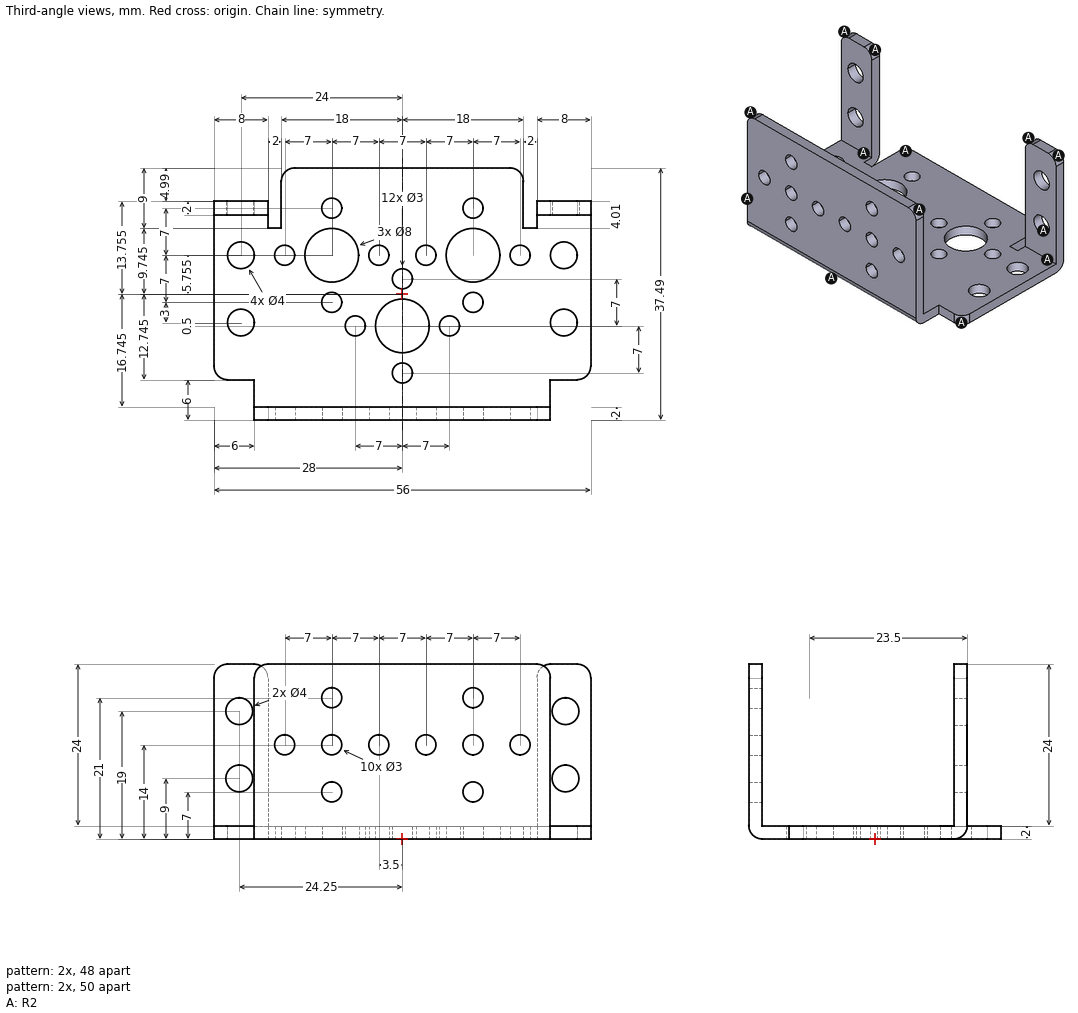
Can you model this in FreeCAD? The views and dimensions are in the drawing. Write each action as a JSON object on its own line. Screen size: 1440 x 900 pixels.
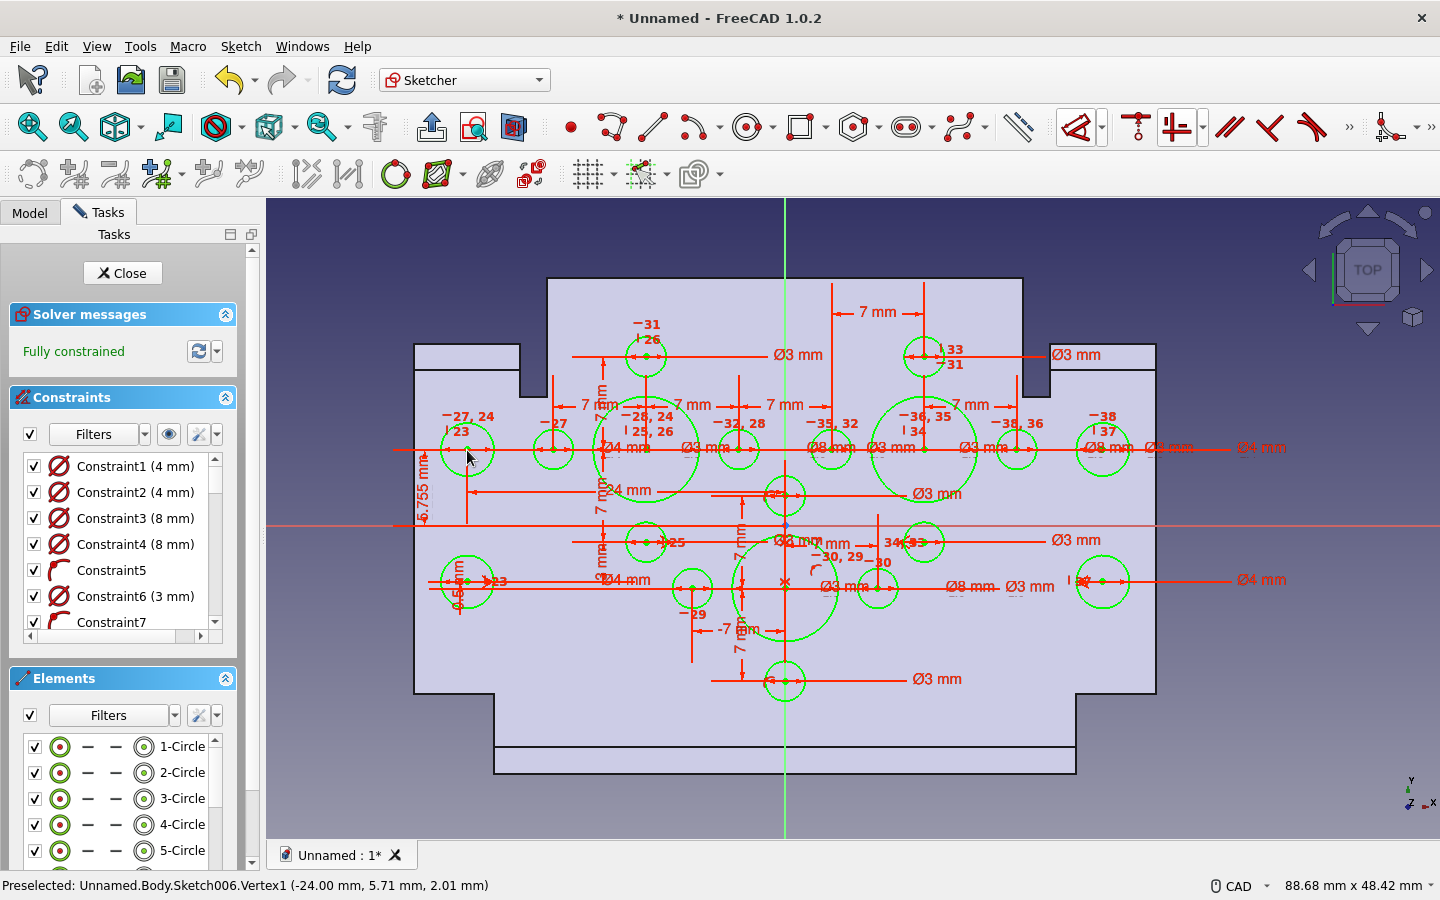
{"action": "left_click", "coordinate": [123, 273]}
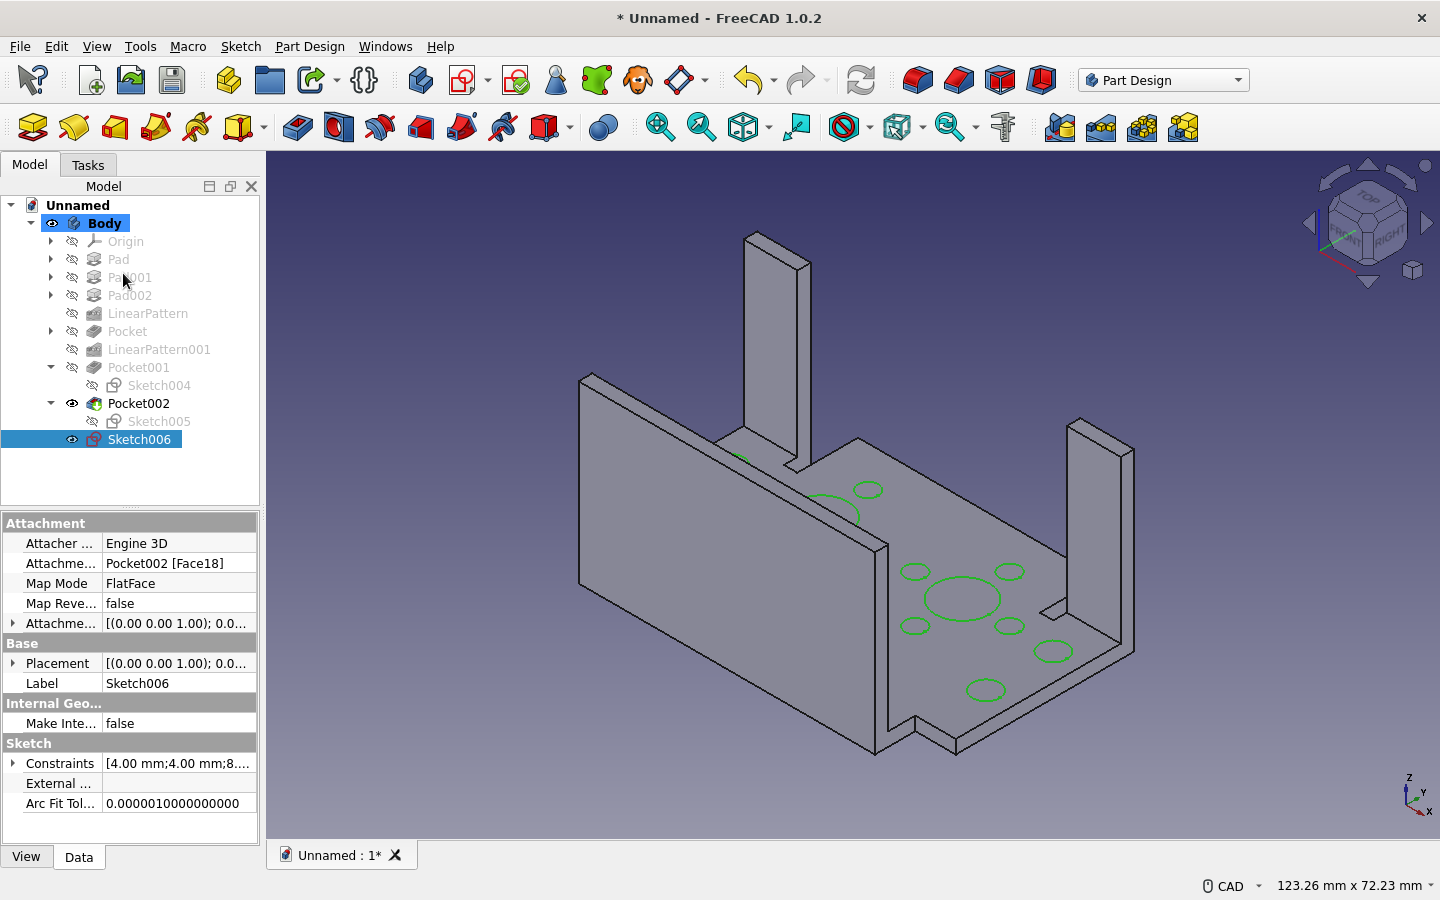
{"action": "left_click", "coordinate": [298, 128]}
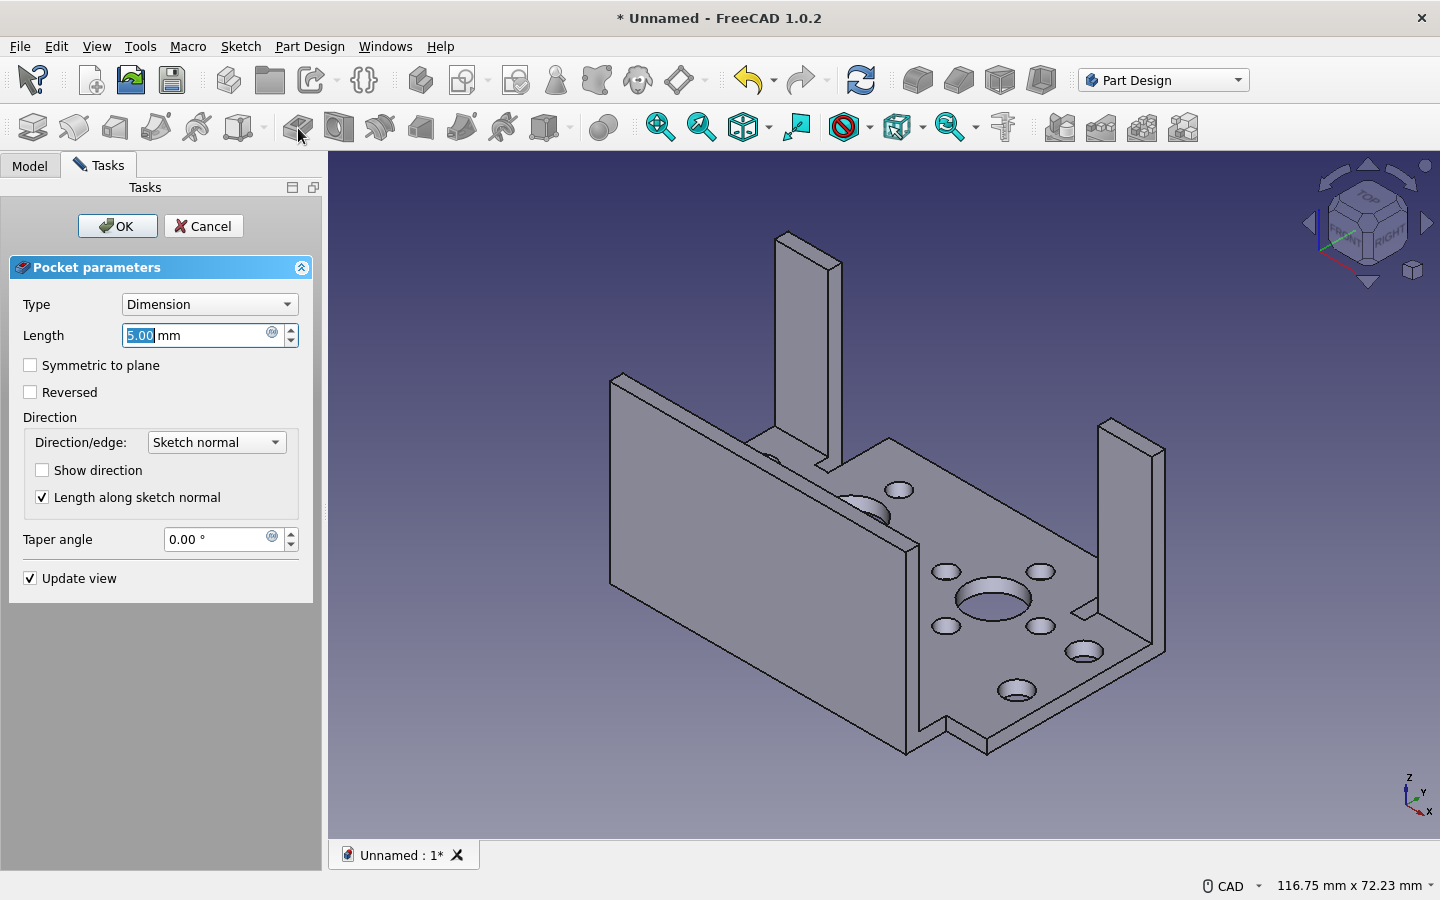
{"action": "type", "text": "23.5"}
{"action": "key", "text": "Tab"}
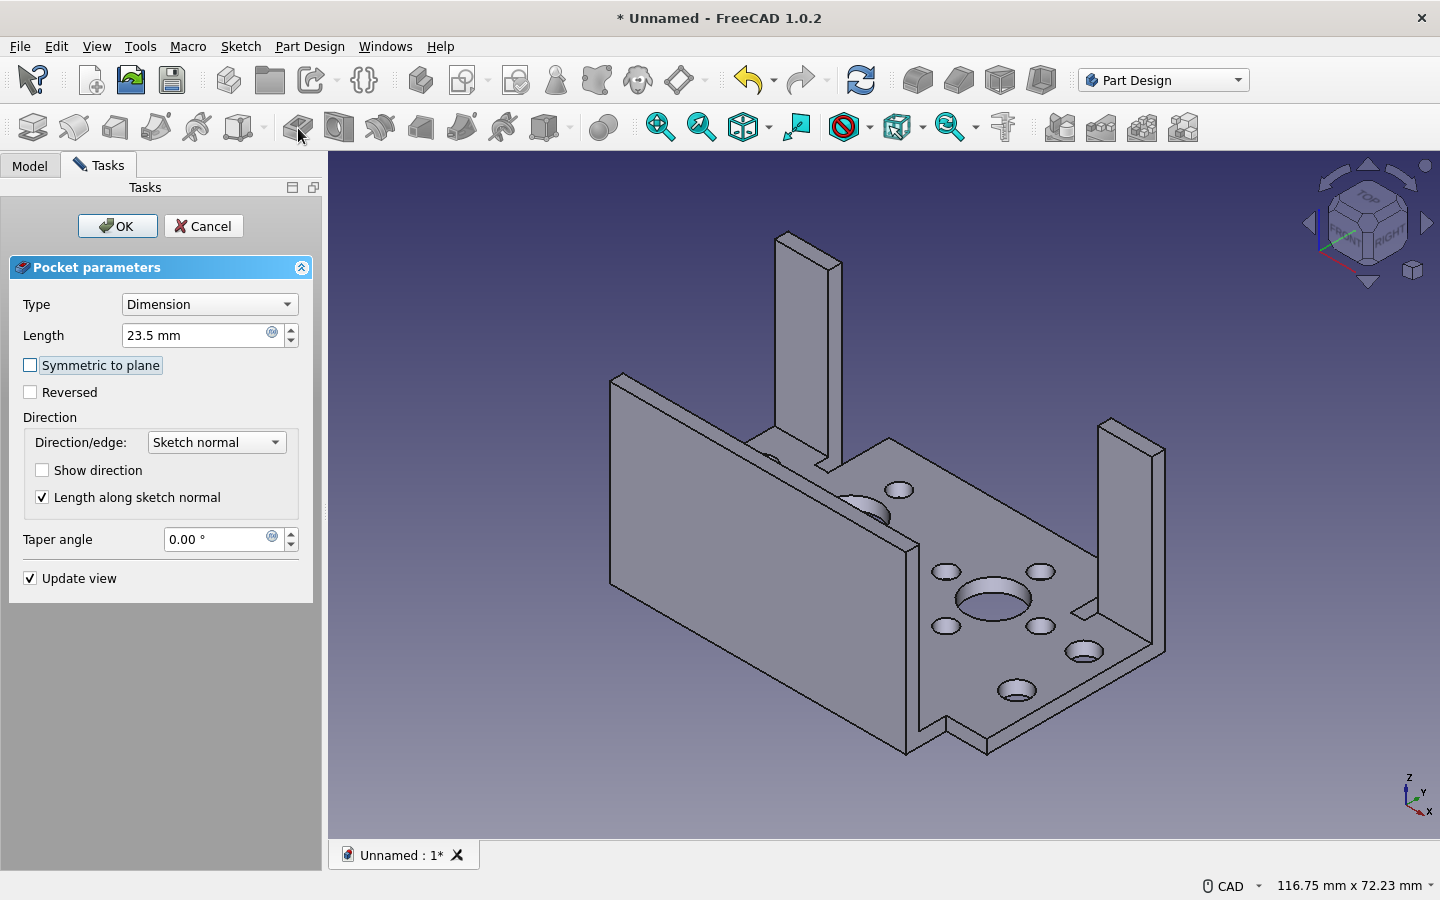
{"action": "left_click", "coordinate": [118, 226]}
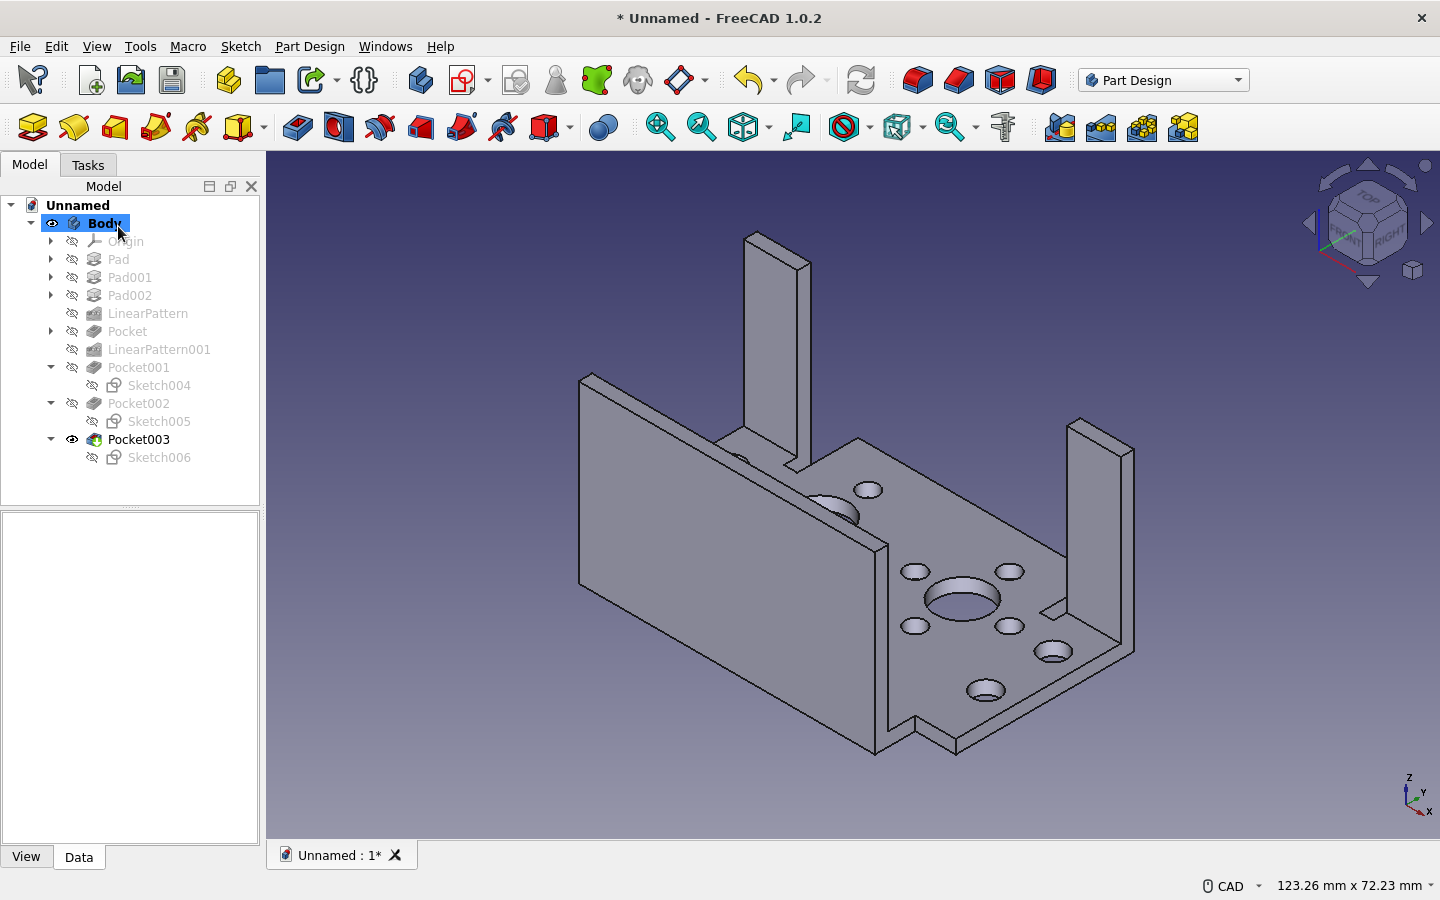
{"action": "key", "text": "4"}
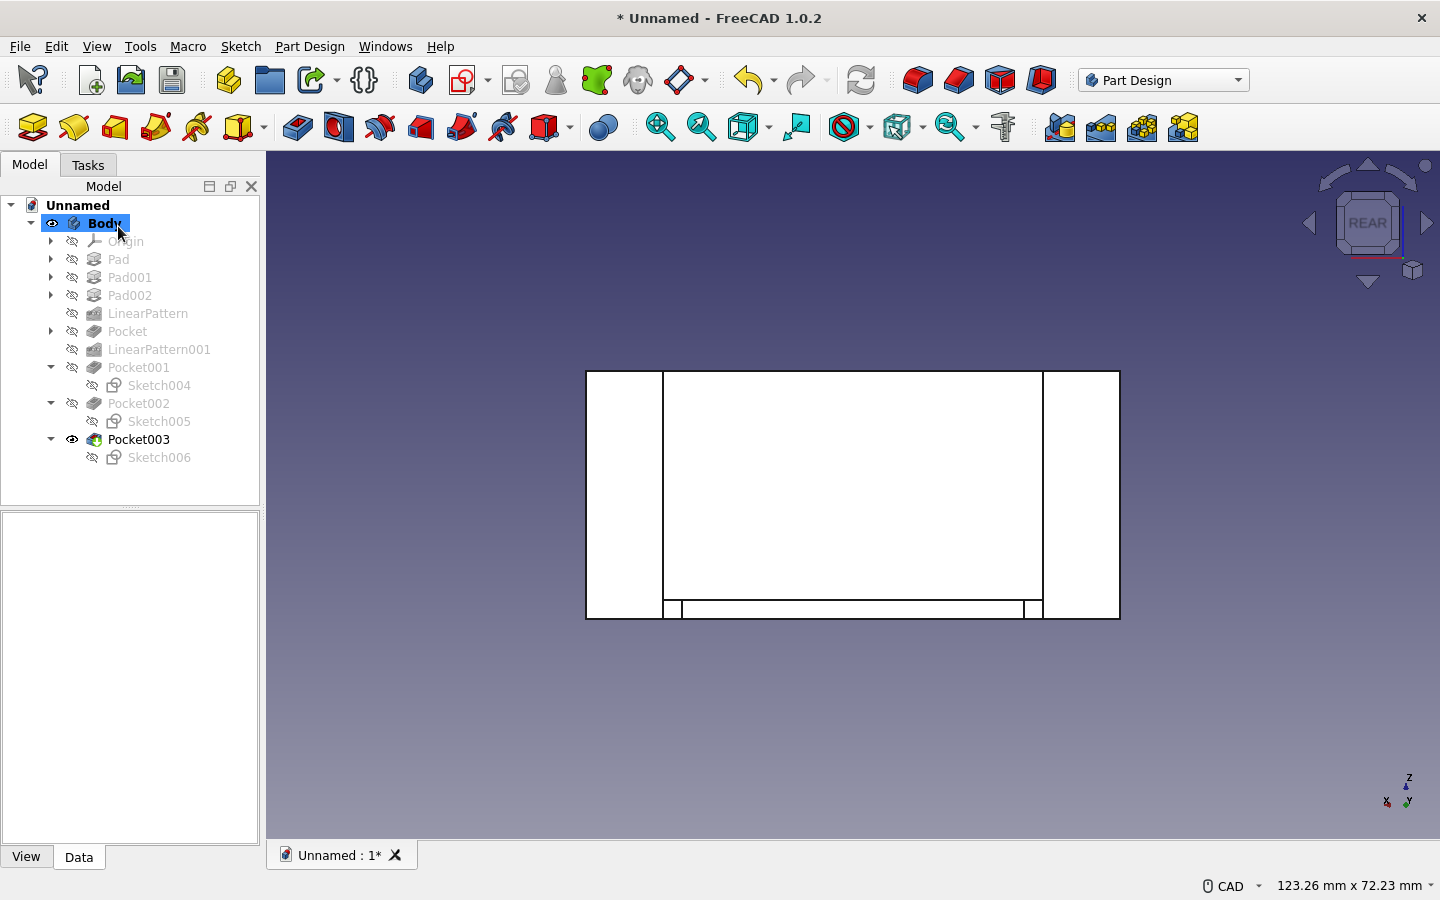
{"action": "left_click", "coordinate": [793, 484]}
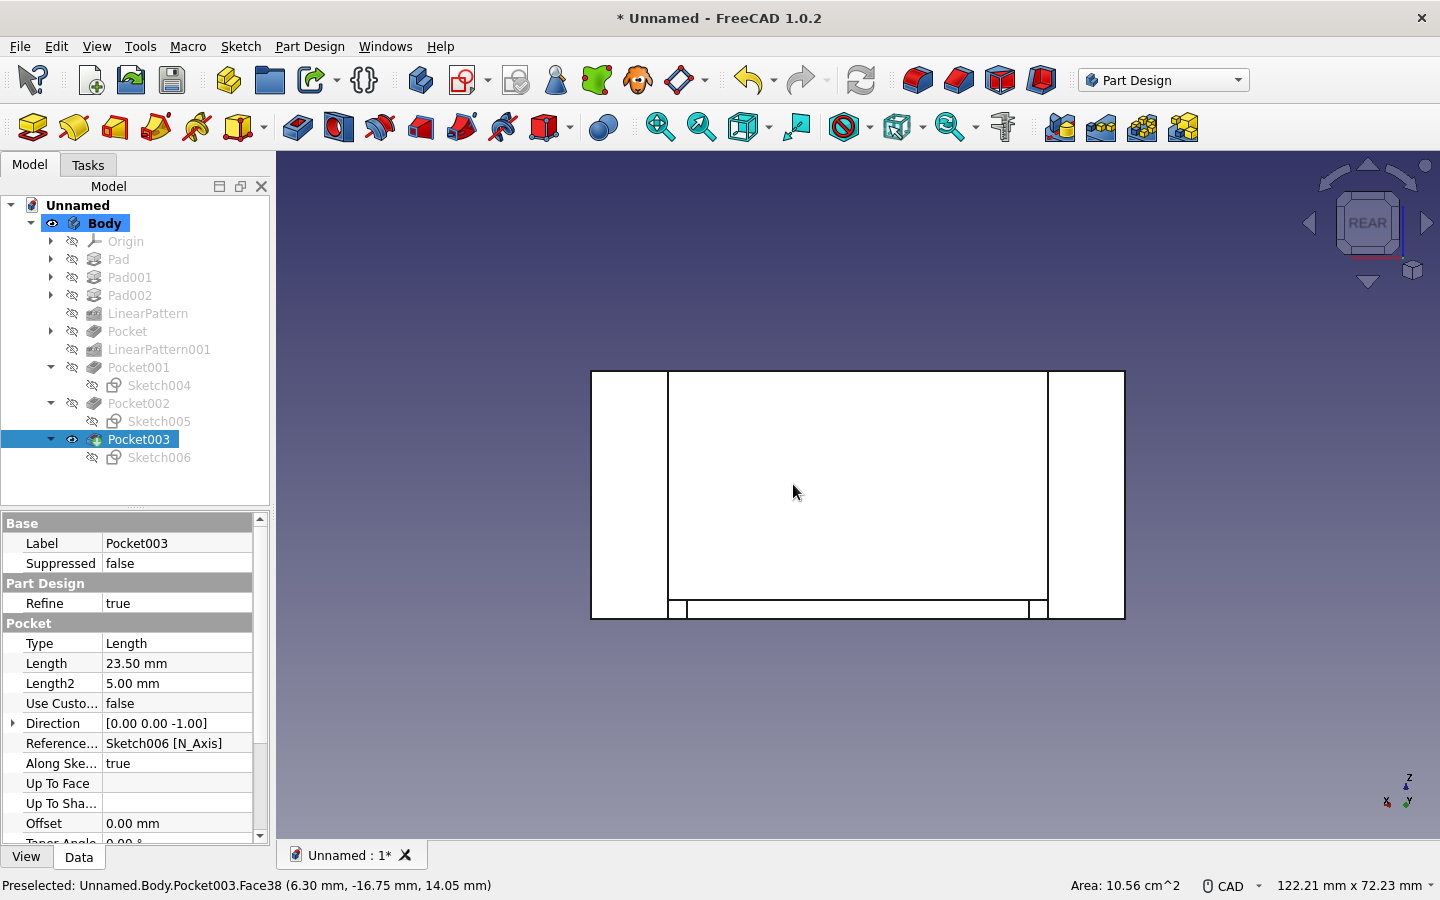
{"action": "left_click", "coordinate": [462, 80]}